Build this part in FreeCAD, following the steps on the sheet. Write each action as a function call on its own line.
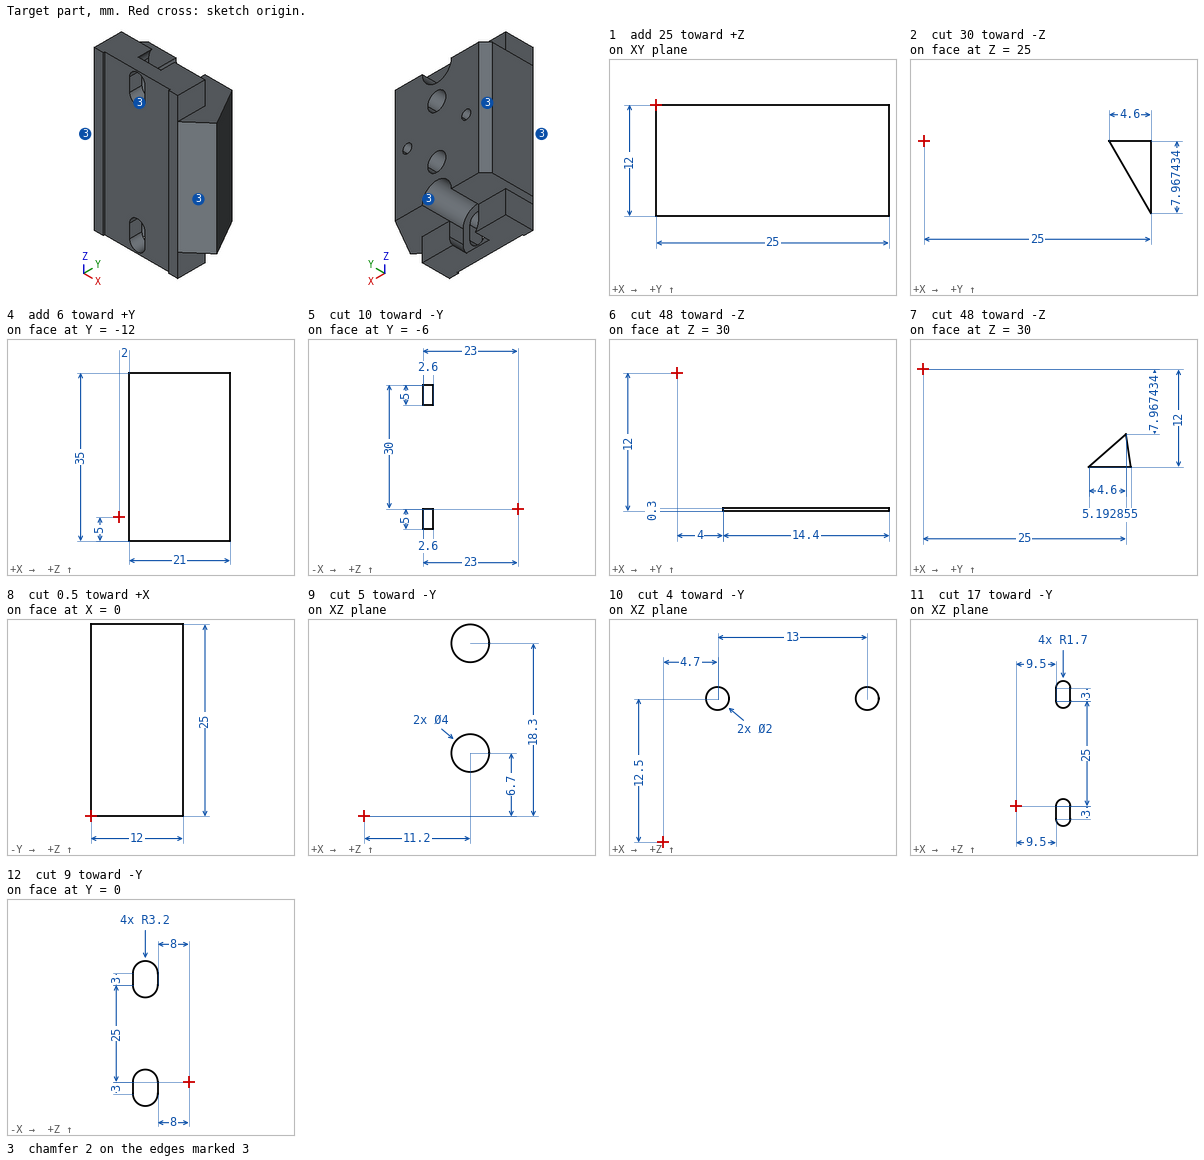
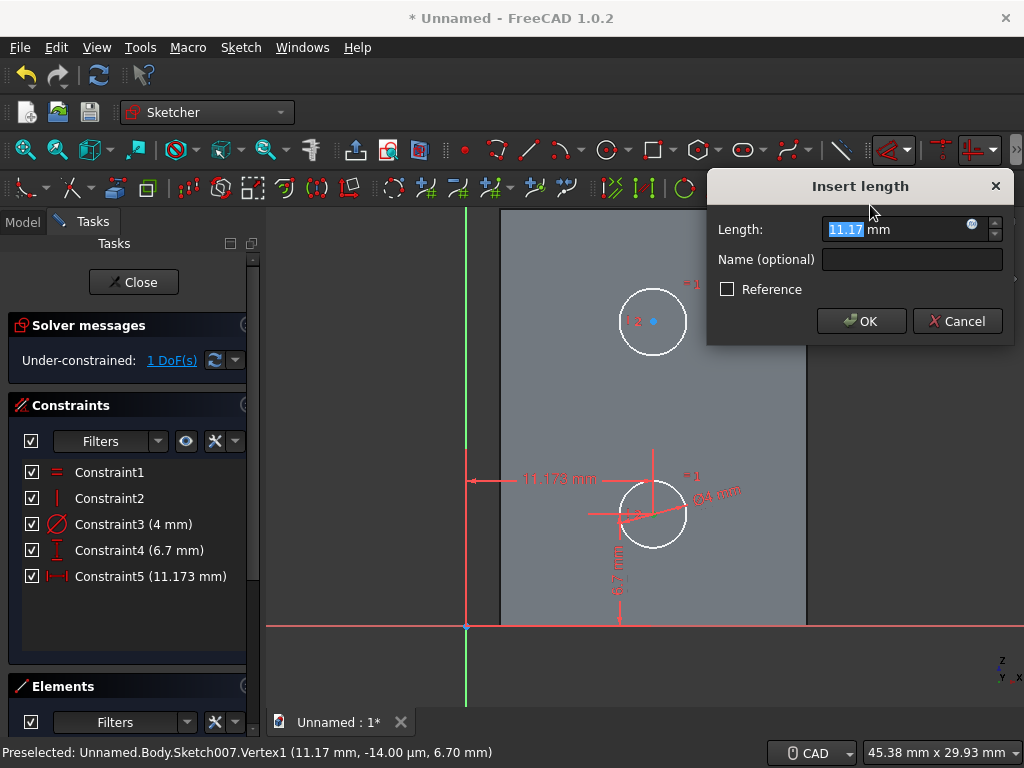
text(11.2)
key(Return)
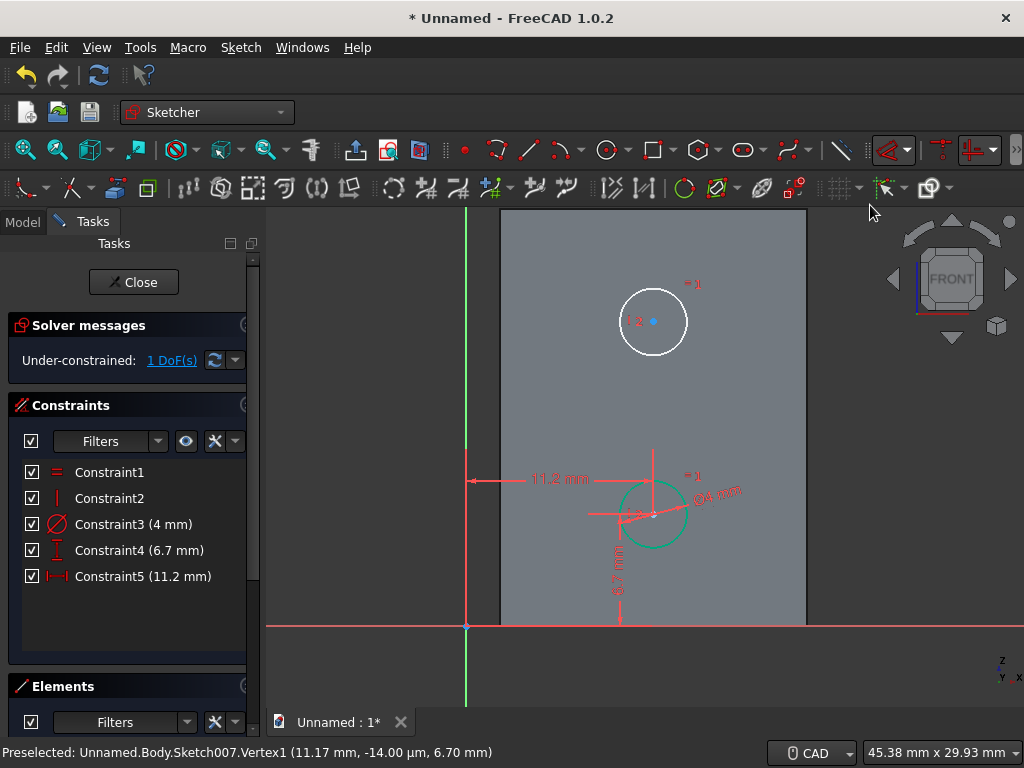
click(653, 322)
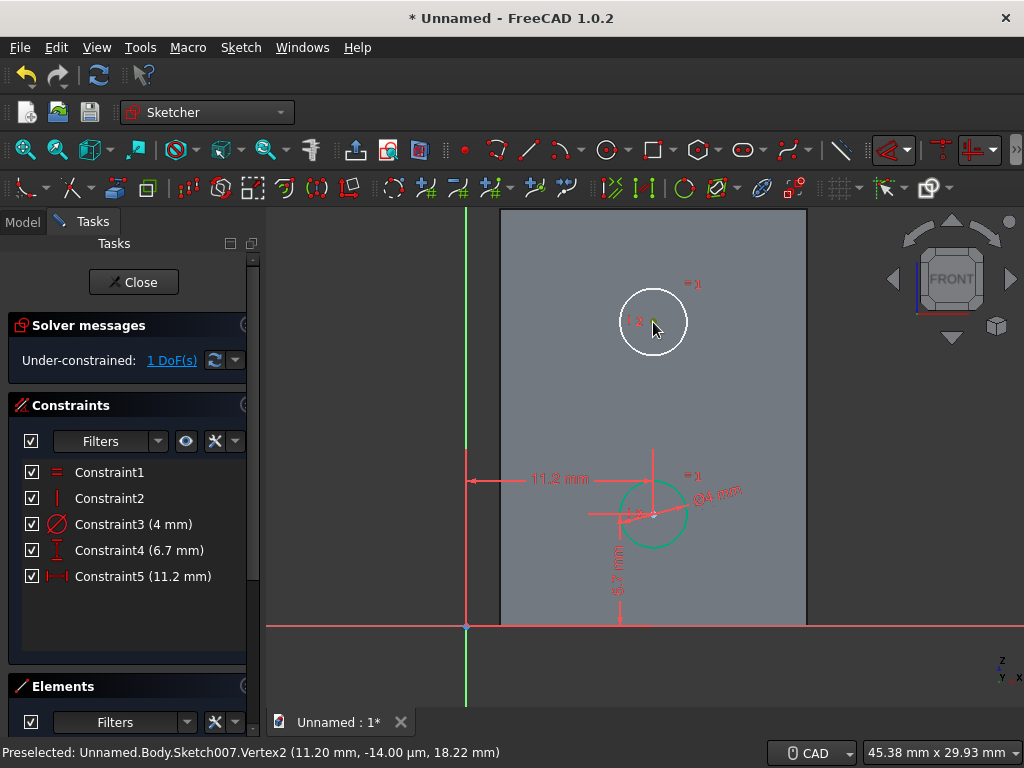
click(910, 150)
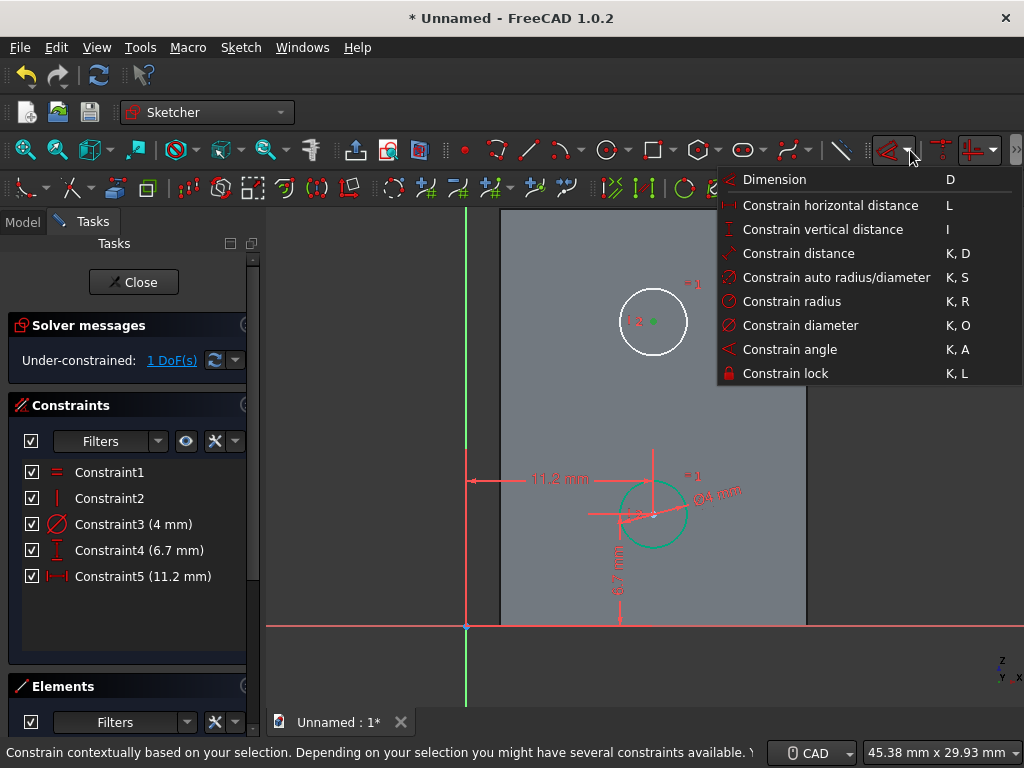
click(870, 229)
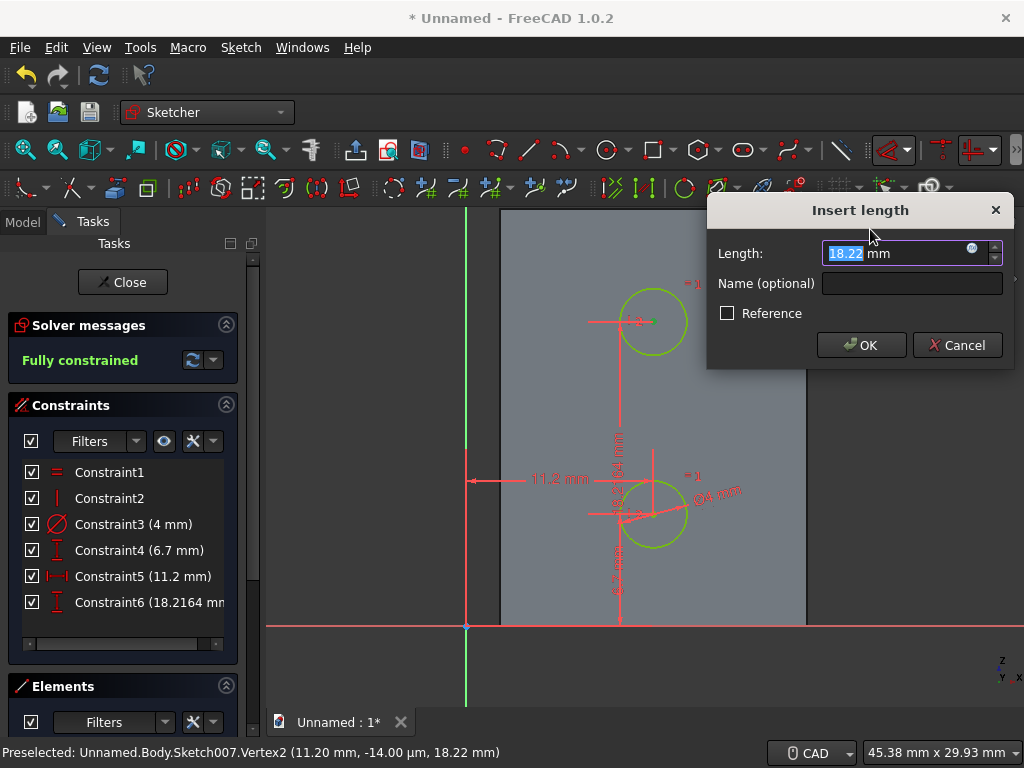
text(18.3)
key(Return)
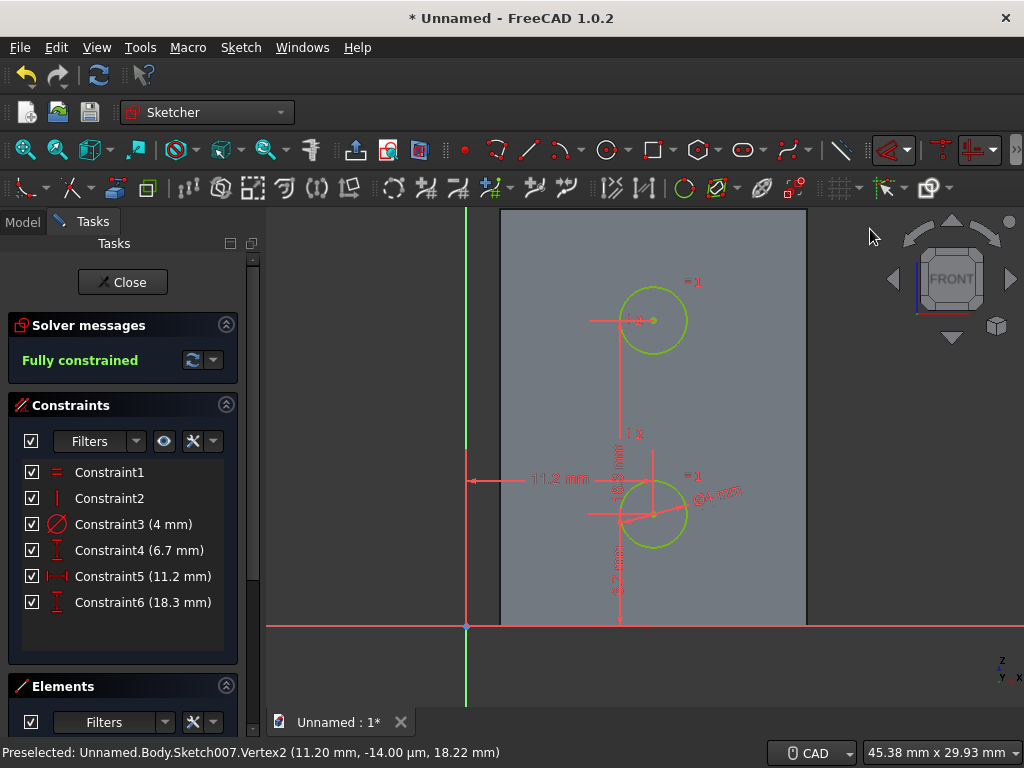
click(123, 282)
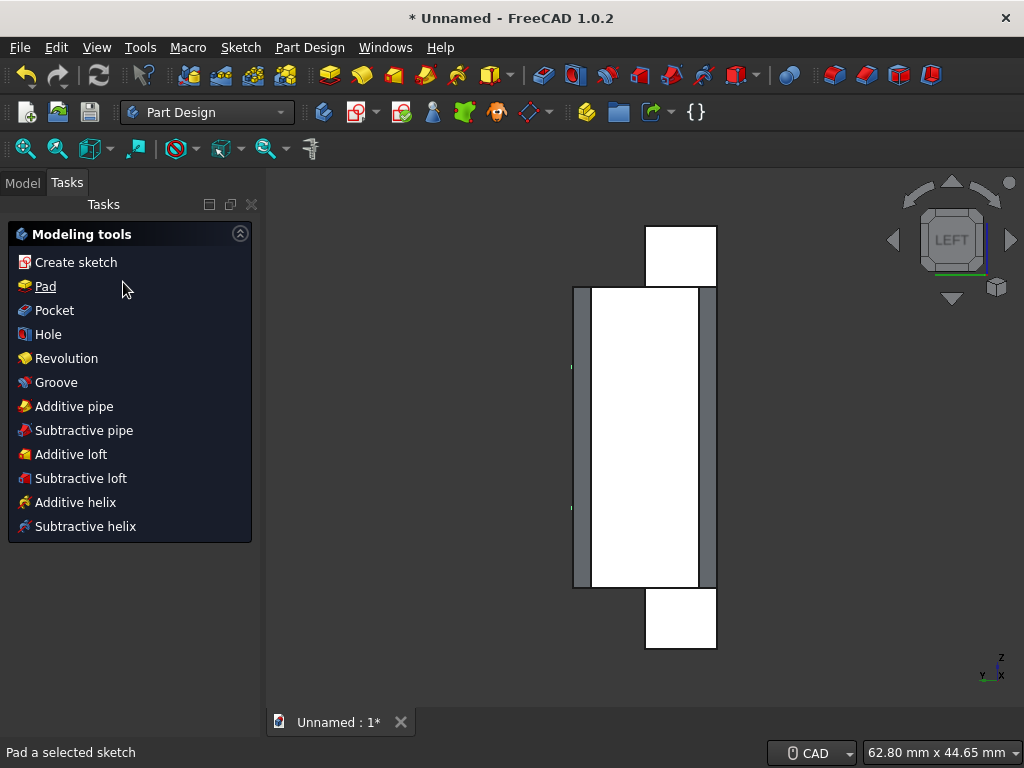
click(544, 76)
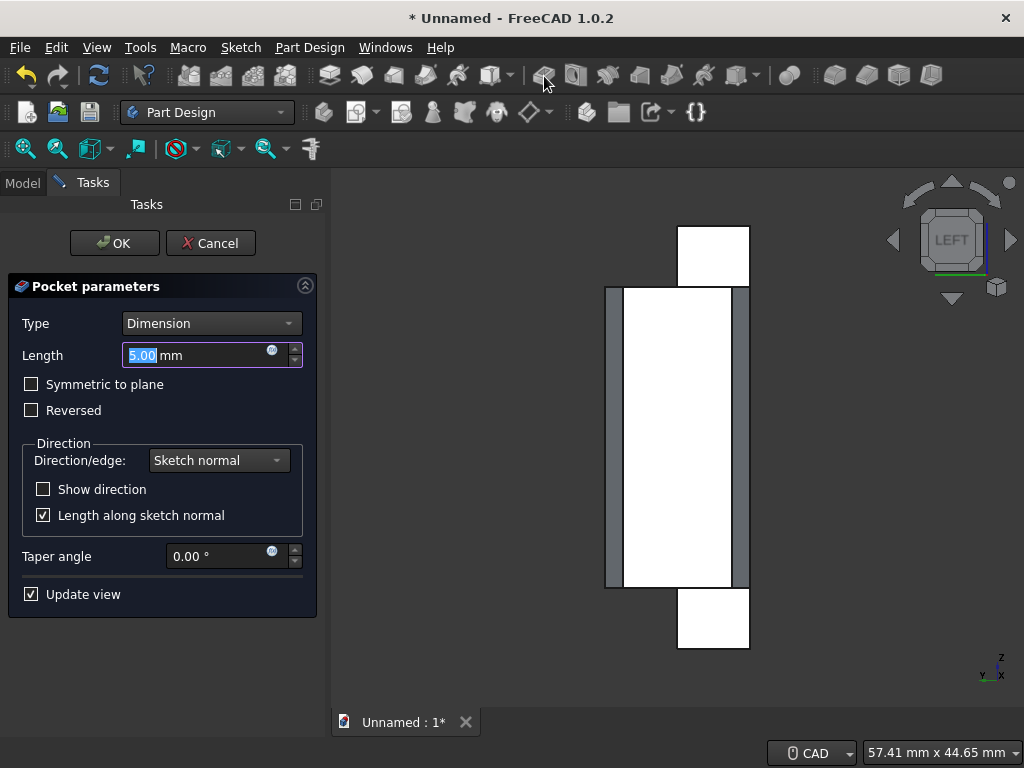
text(5)
key(Tab)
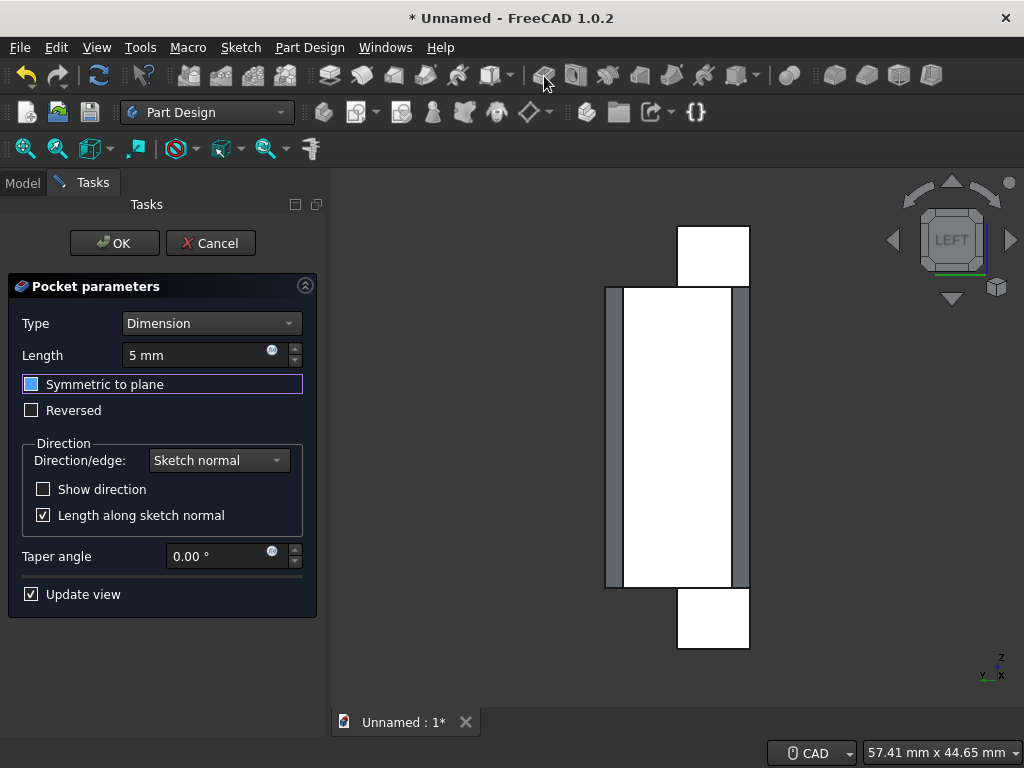
click(30, 410)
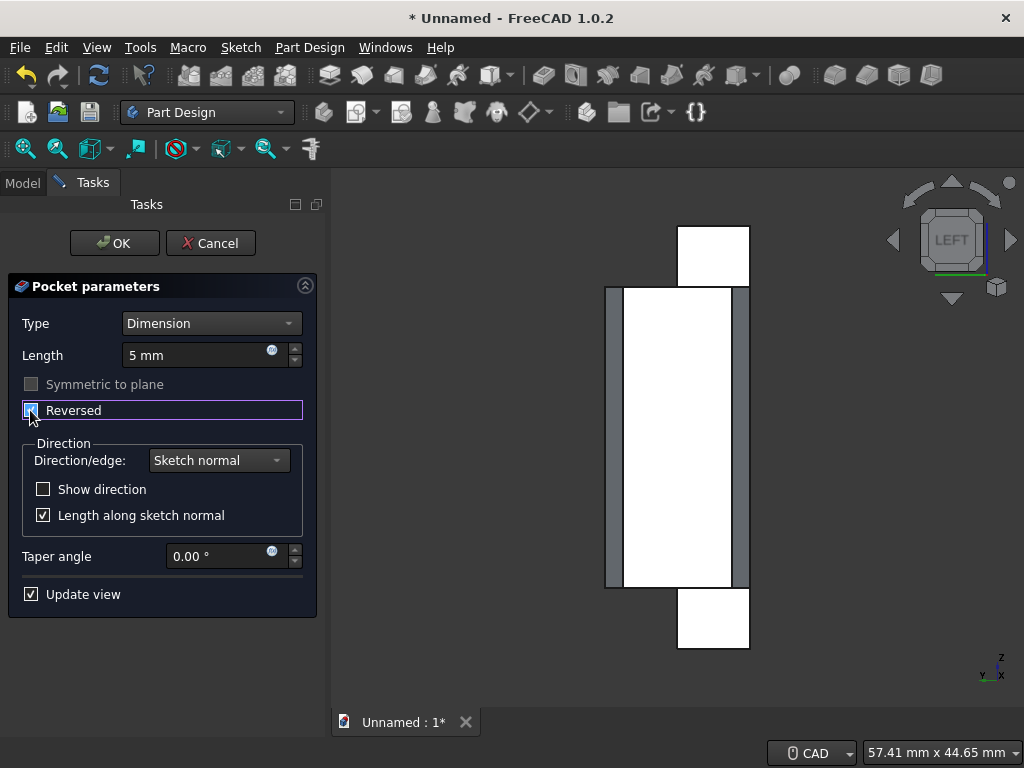
click(115, 243)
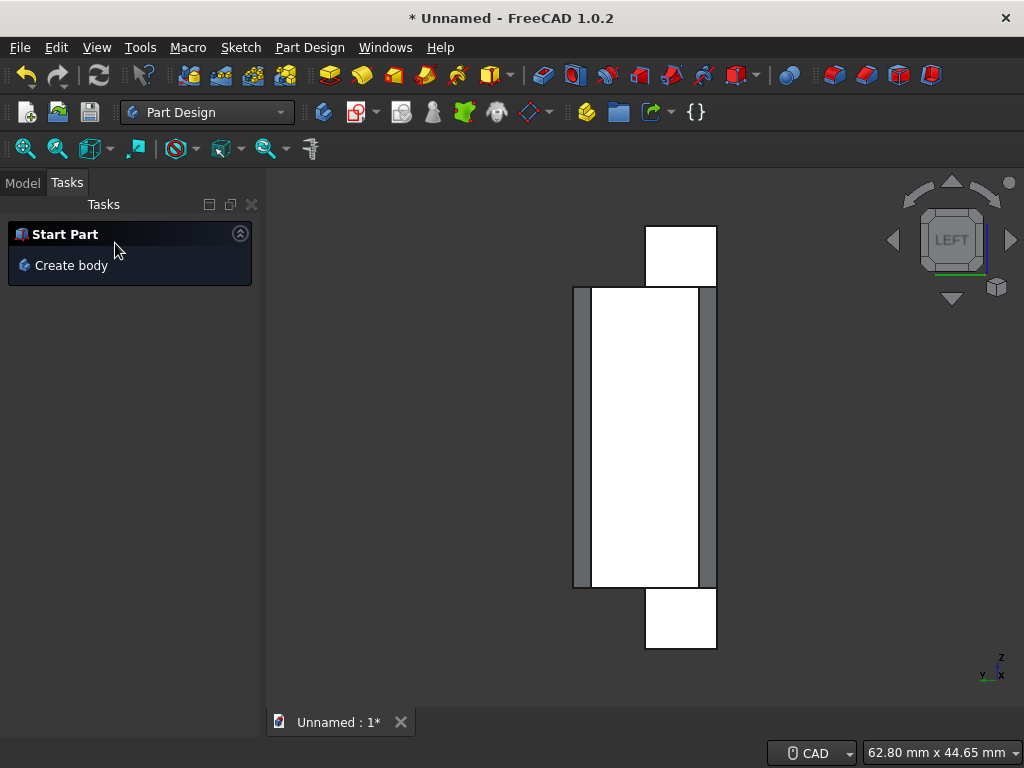
click(356, 112)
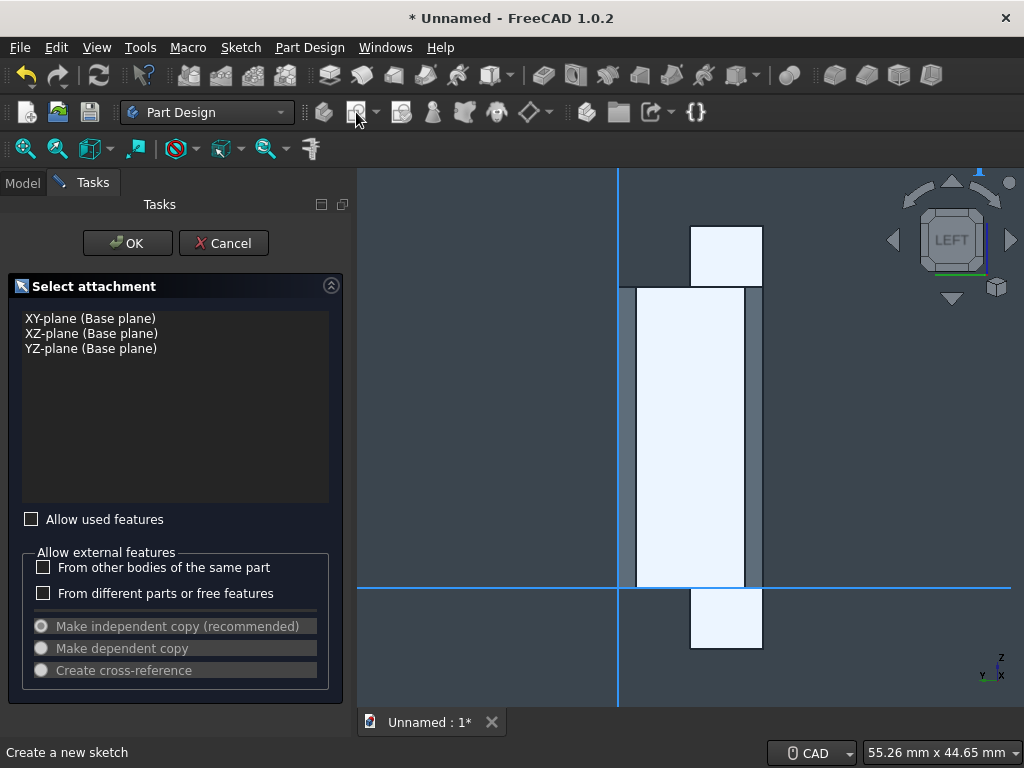
click(82, 334)